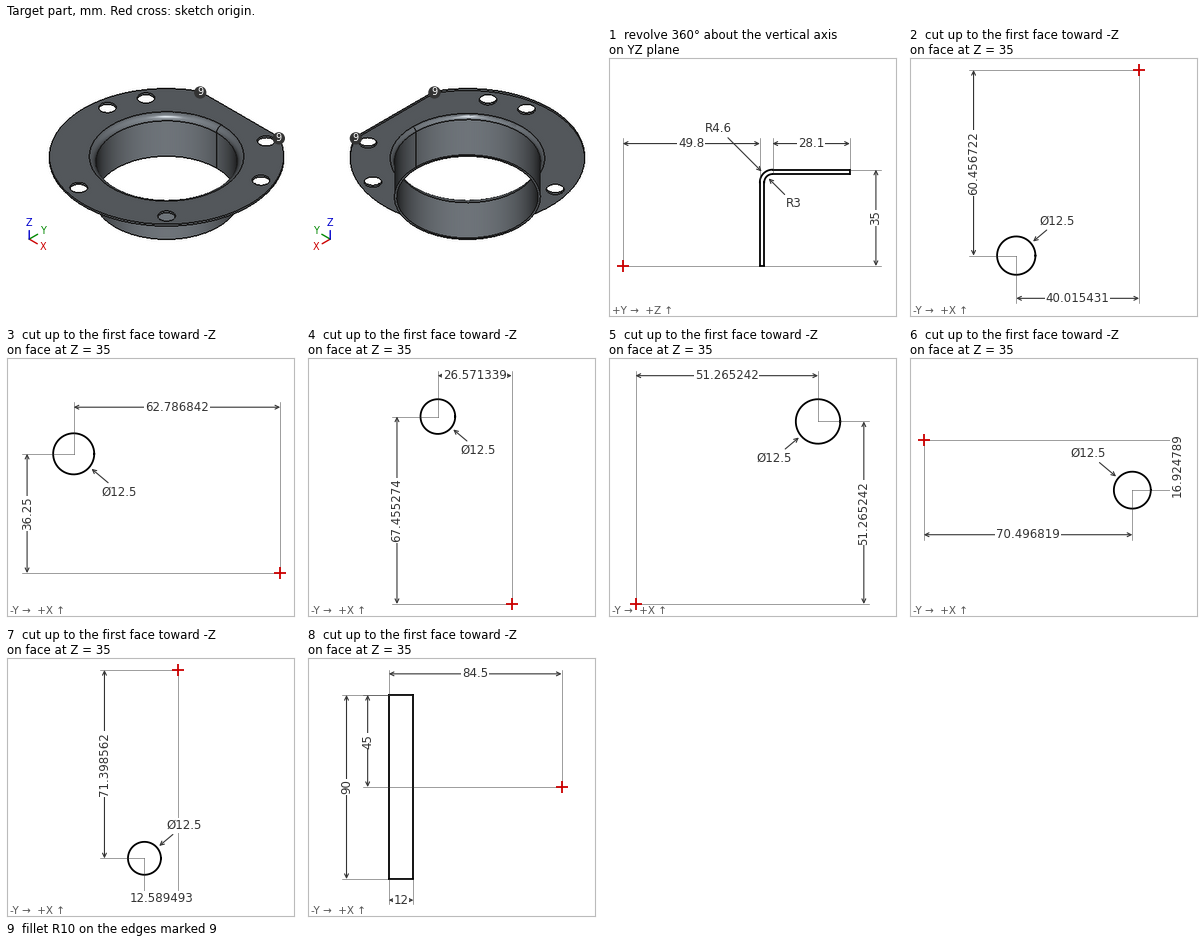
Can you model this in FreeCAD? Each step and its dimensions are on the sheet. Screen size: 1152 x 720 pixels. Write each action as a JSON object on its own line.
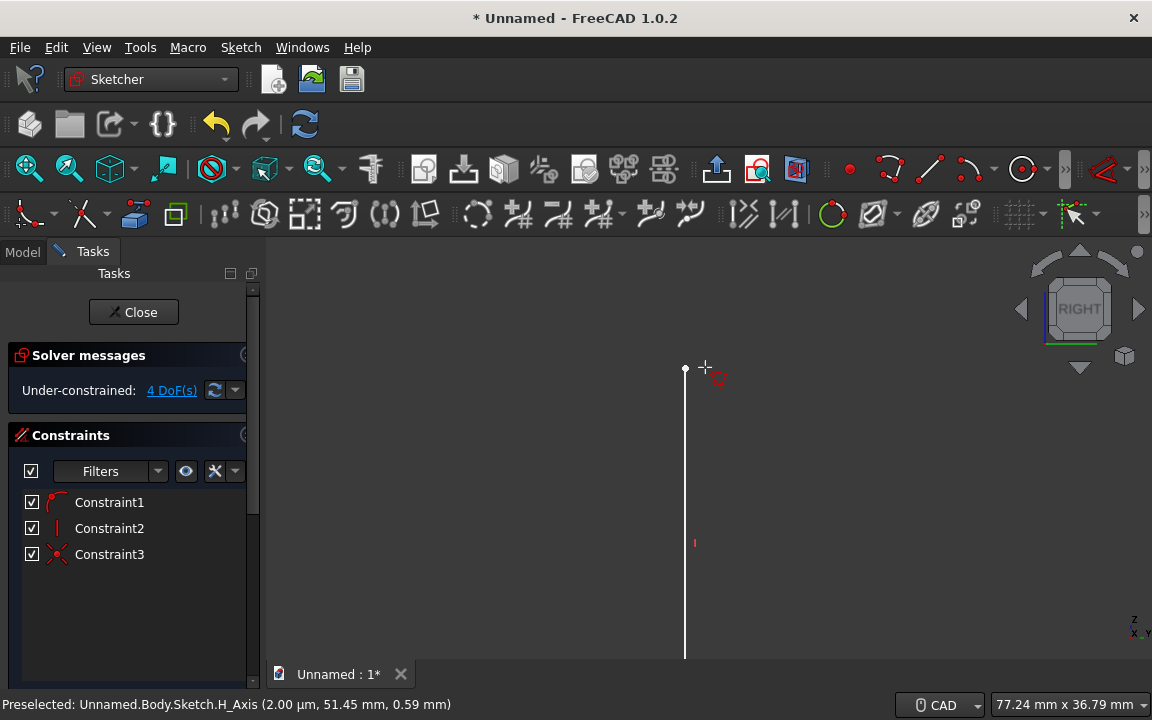
{"action": "left_click", "coordinate": [704, 367]}
{"action": "right_click", "coordinate": [704, 367]}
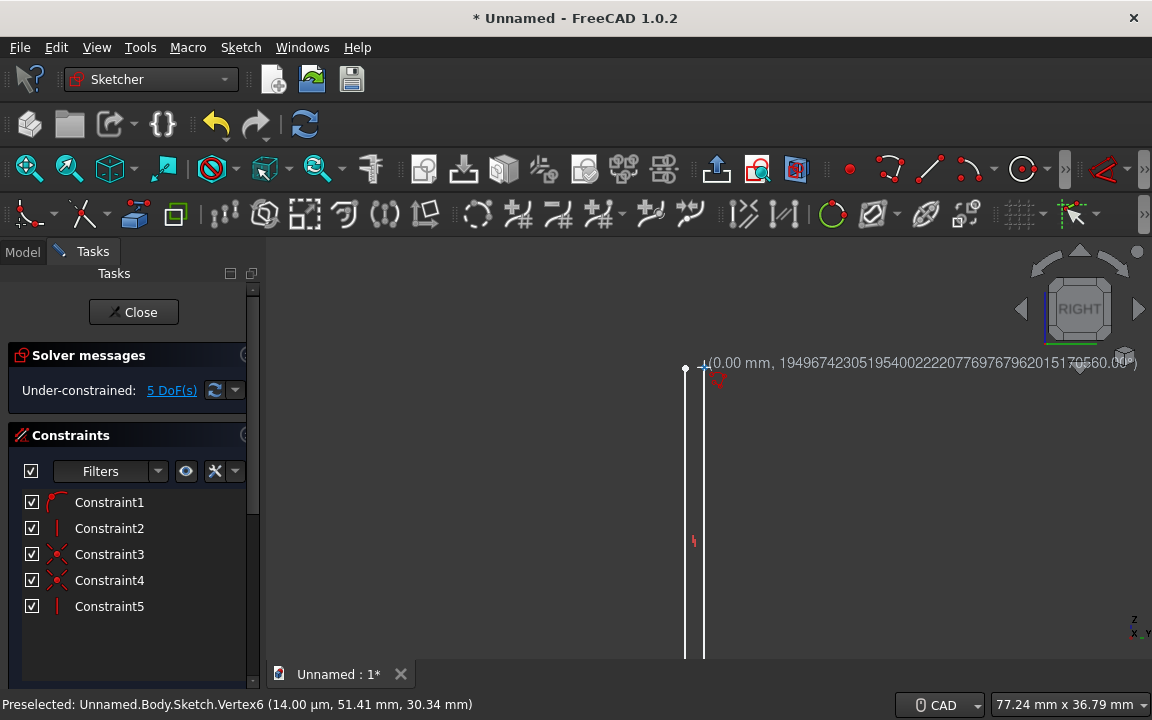
{"action": "left_click", "coordinate": [738, 333]}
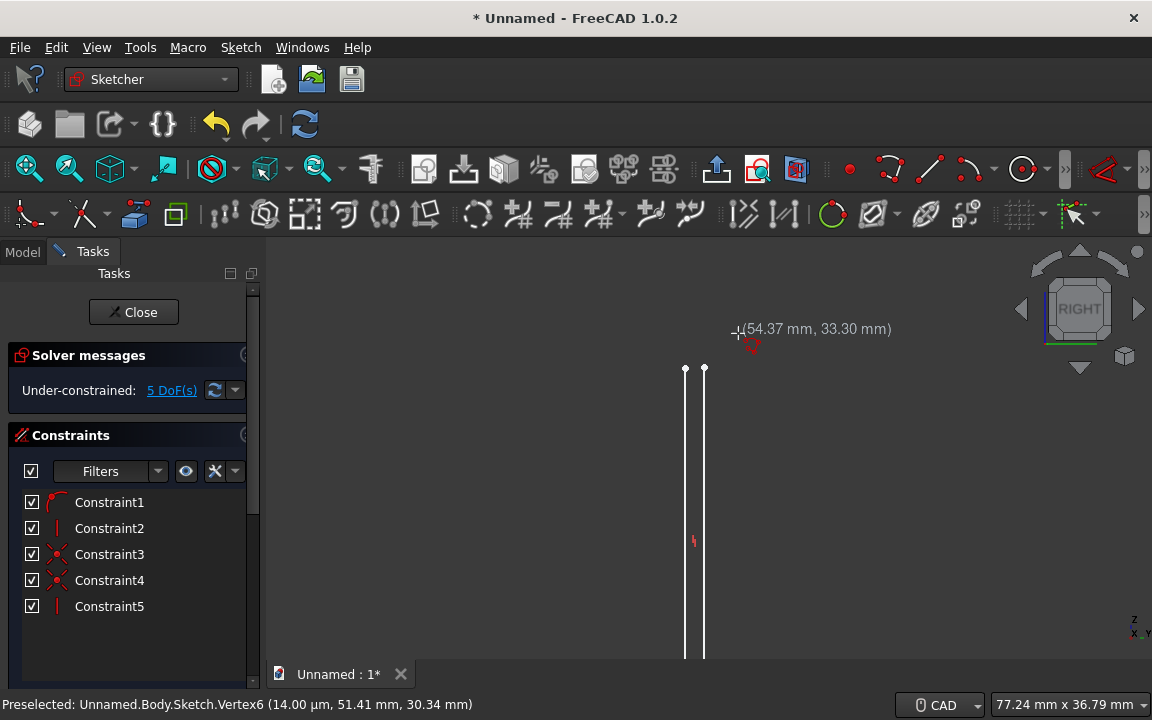
{"action": "scroll", "coordinate": [705, 366], "scroll_direction": "down", "scroll_amount": 3}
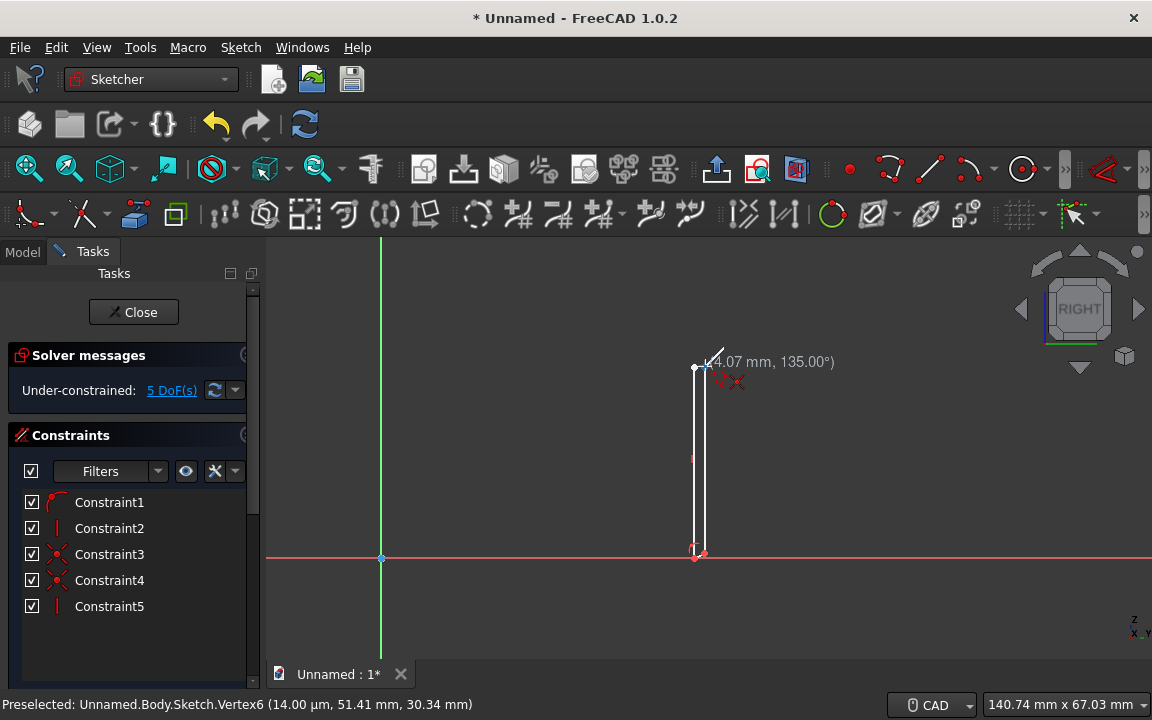
{"action": "left_click", "coordinate": [900, 348]}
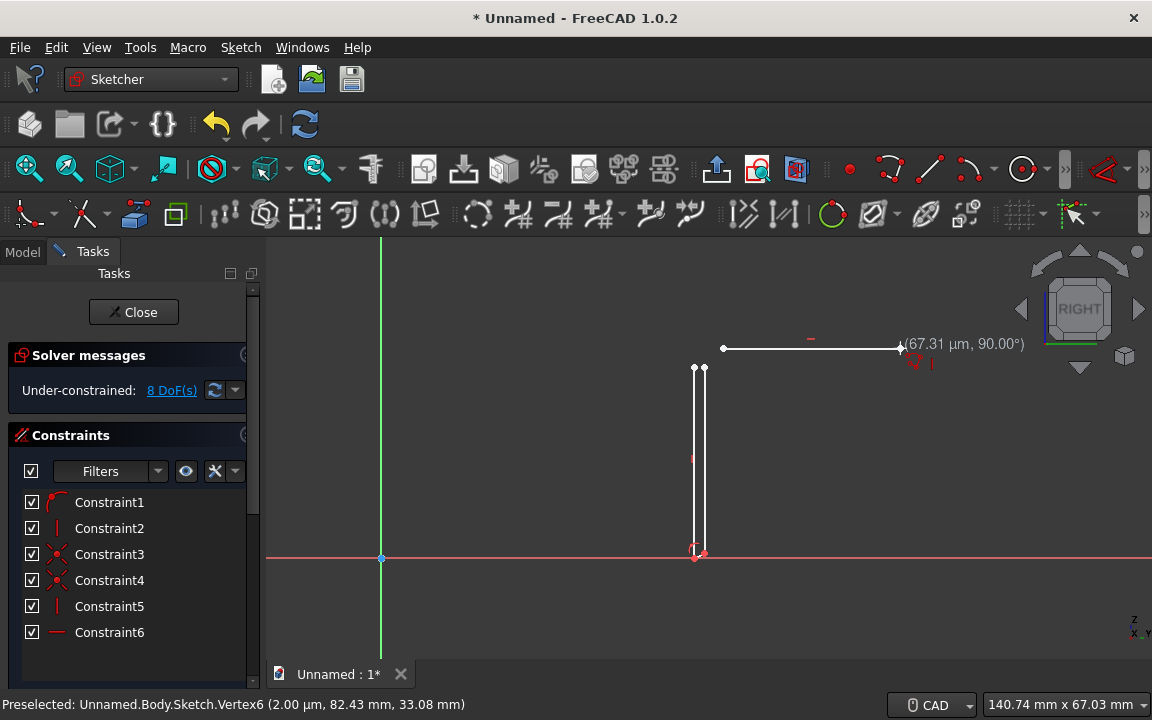
{"action": "scroll", "coordinate": [900, 338], "scroll_direction": "up", "scroll_amount": 3}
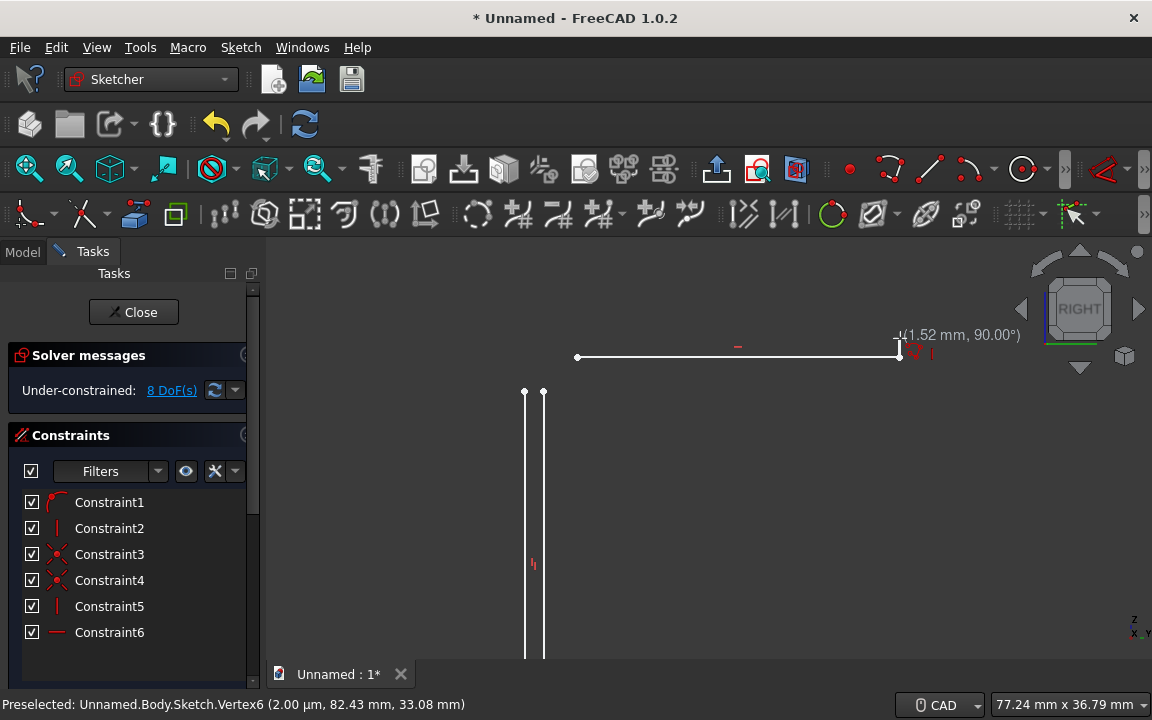
{"action": "left_click", "coordinate": [899, 338]}
{"action": "left_click", "coordinate": [578, 338]}
{"action": "right_click", "coordinate": [578, 338]}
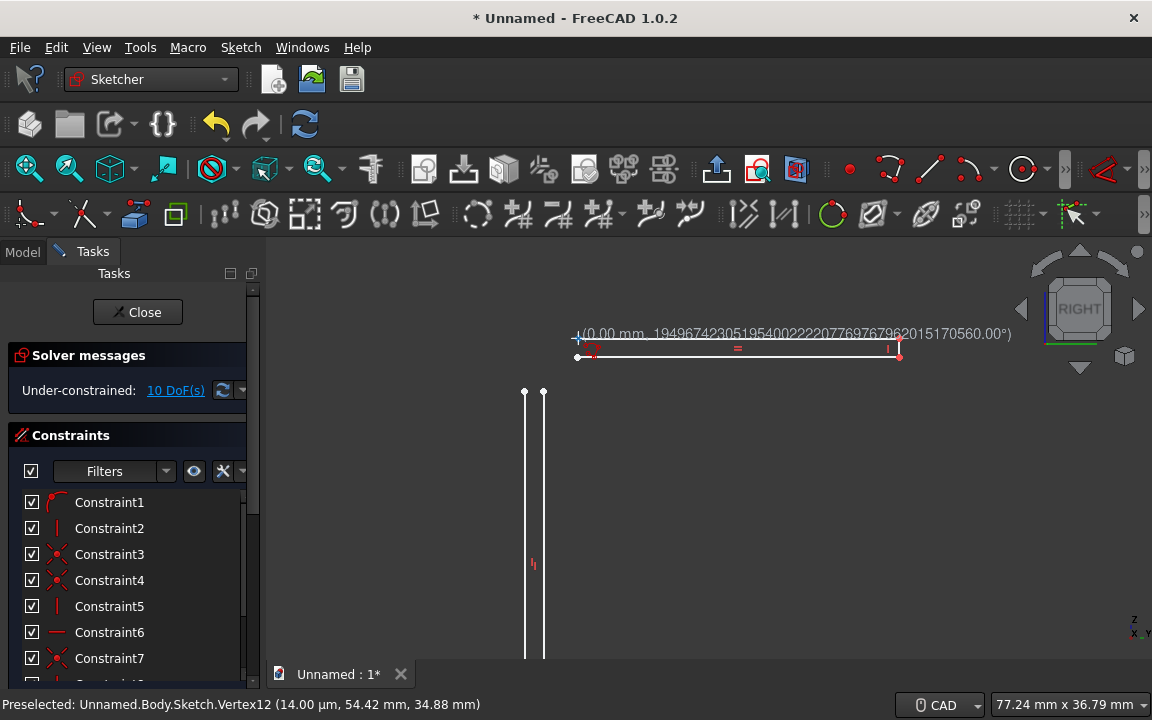
{"action": "left_click", "coordinate": [996, 170]}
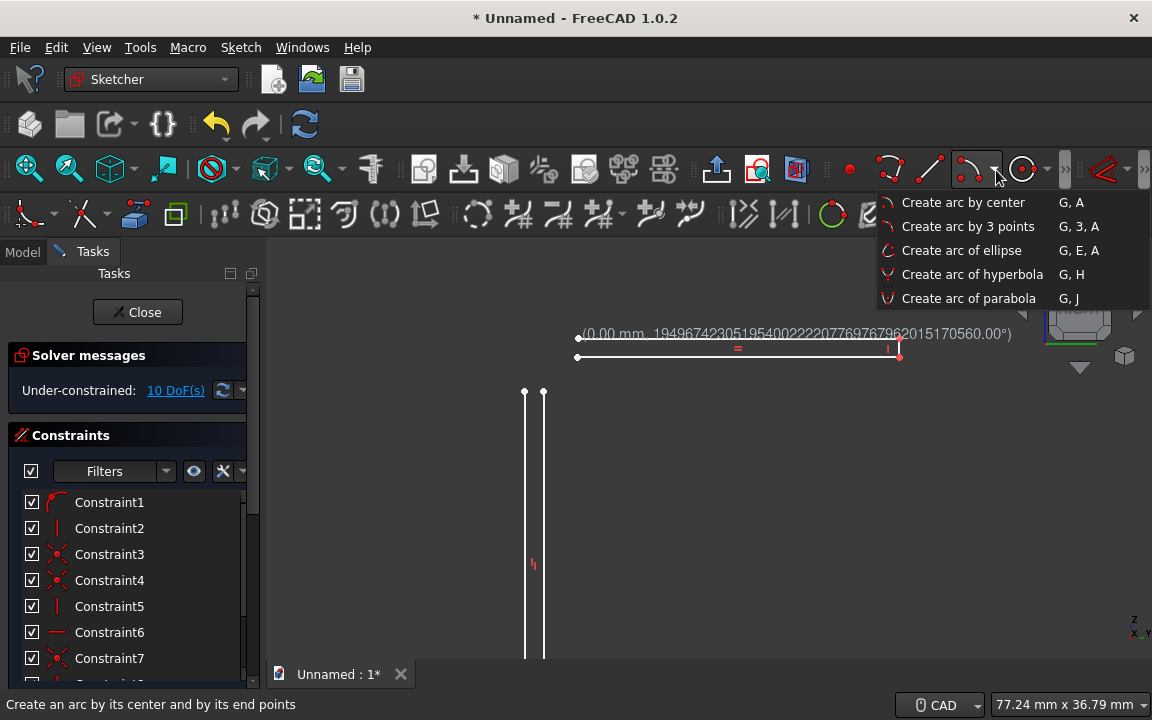
{"action": "left_click", "coordinate": [1014, 226]}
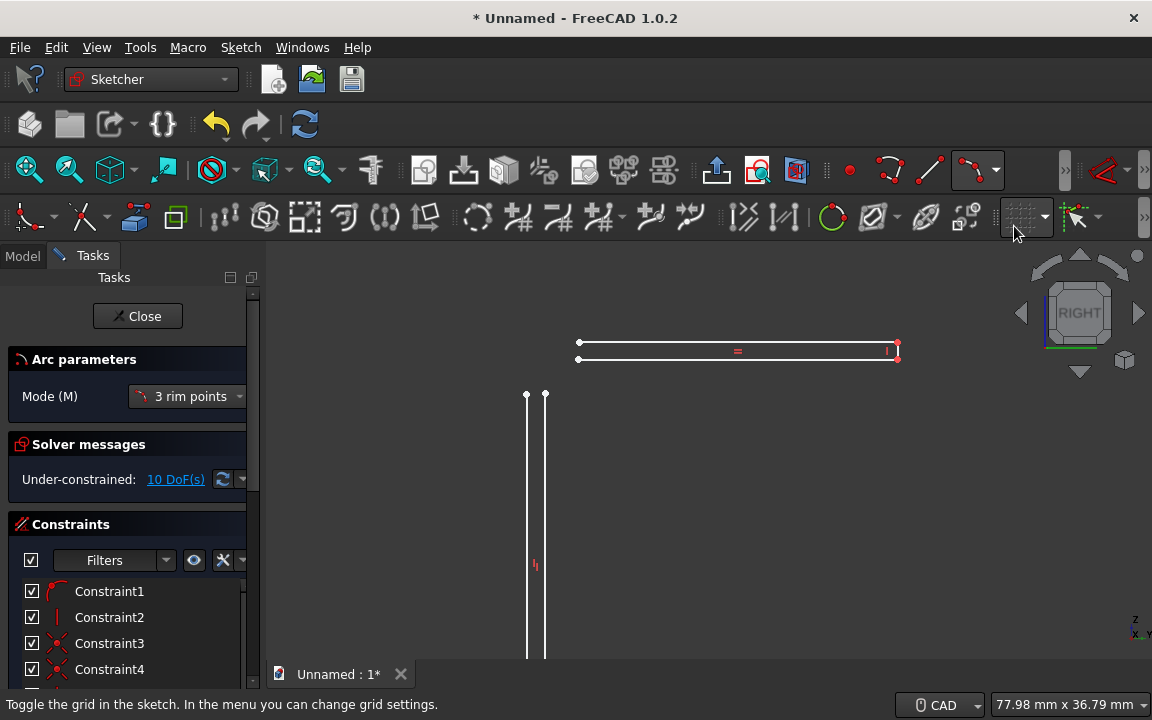
{"action": "left_click", "coordinate": [545, 394]}
{"action": "left_click", "coordinate": [579, 360]}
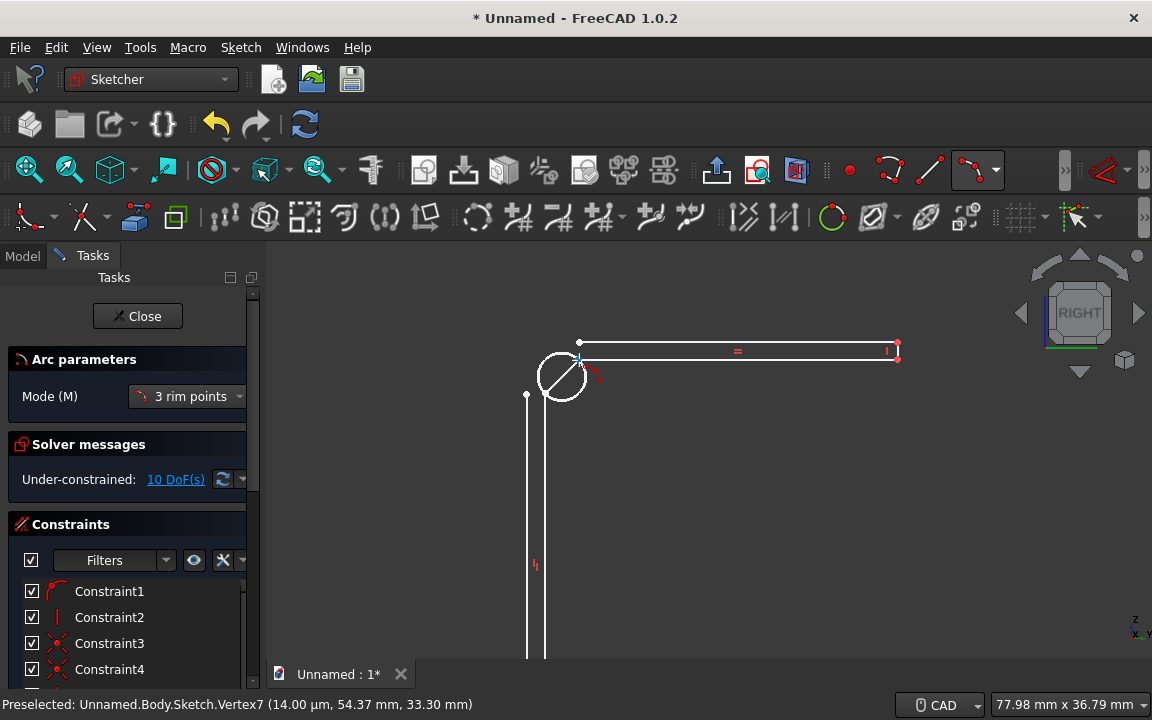
{"action": "scroll", "coordinate": [555, 369], "scroll_direction": "up", "scroll_amount": 3}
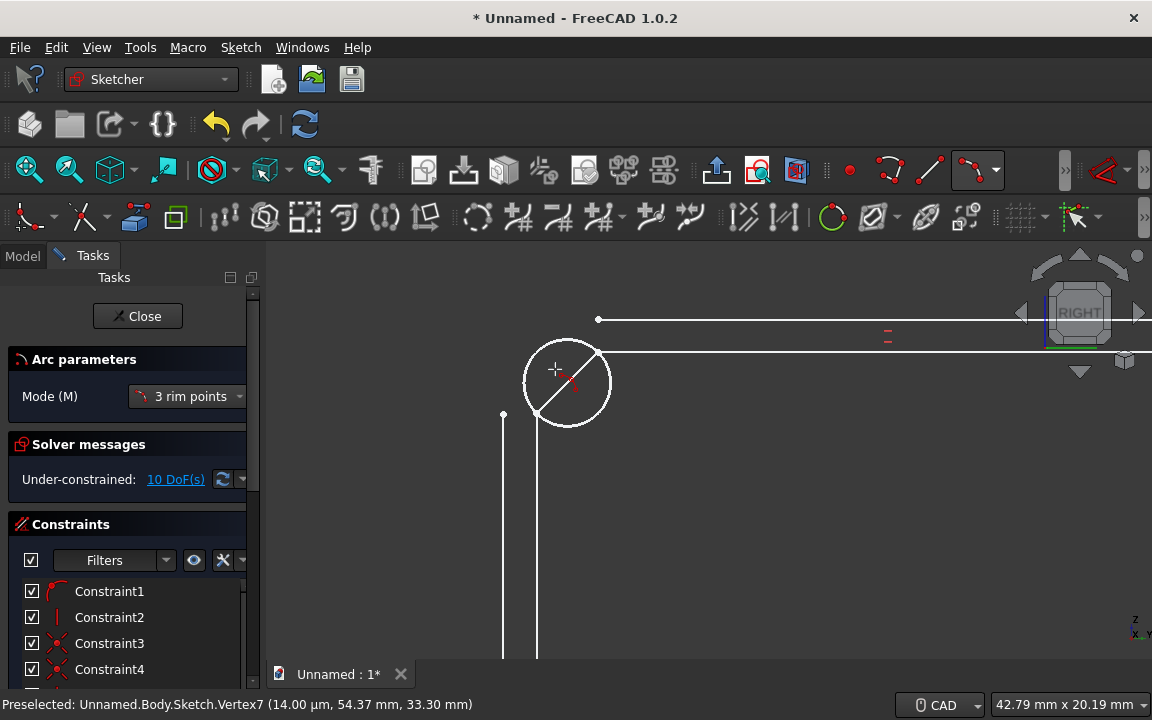
{"action": "left_click", "coordinate": [555, 368]}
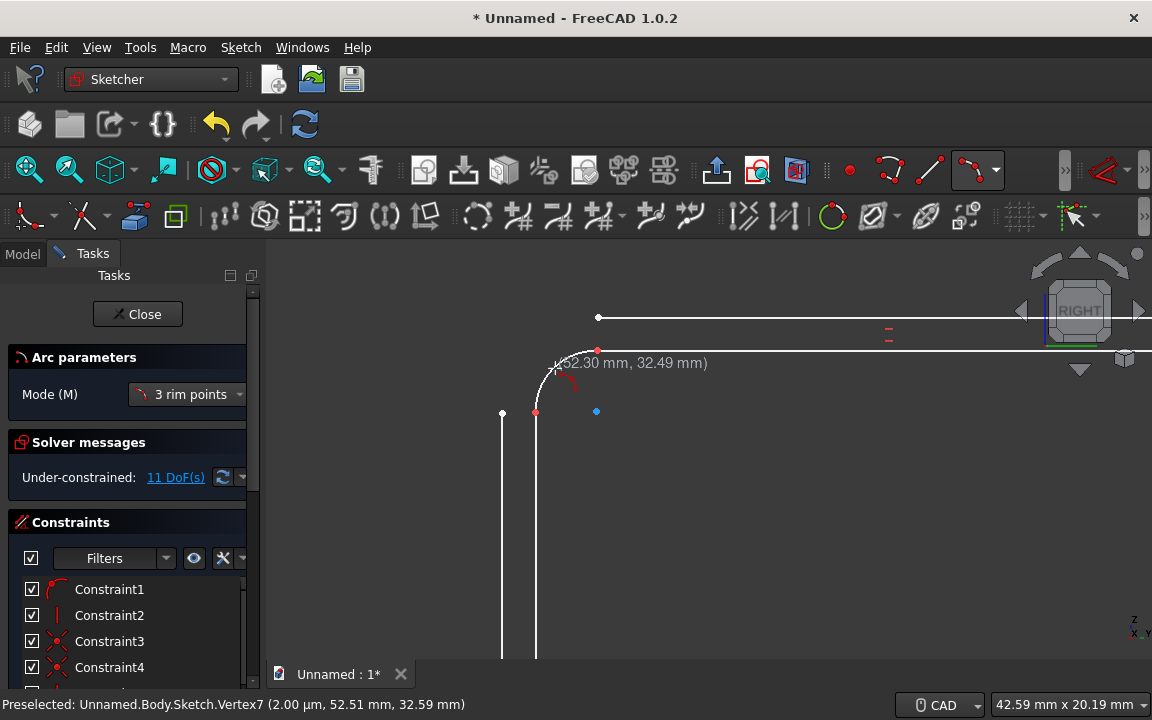
{"action": "left_click", "coordinate": [598, 318]}
{"action": "left_click", "coordinate": [502, 413]}
{"action": "left_click", "coordinate": [530, 343]}
{"action": "key", "text": "Escape"}